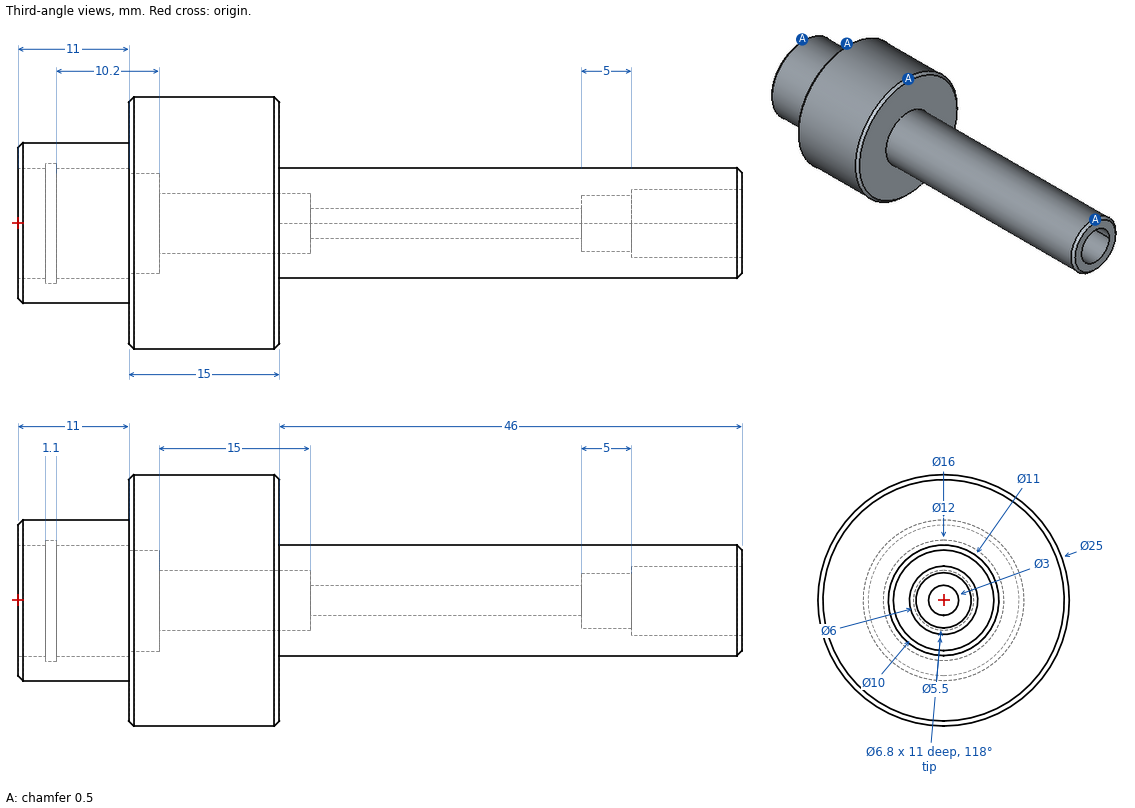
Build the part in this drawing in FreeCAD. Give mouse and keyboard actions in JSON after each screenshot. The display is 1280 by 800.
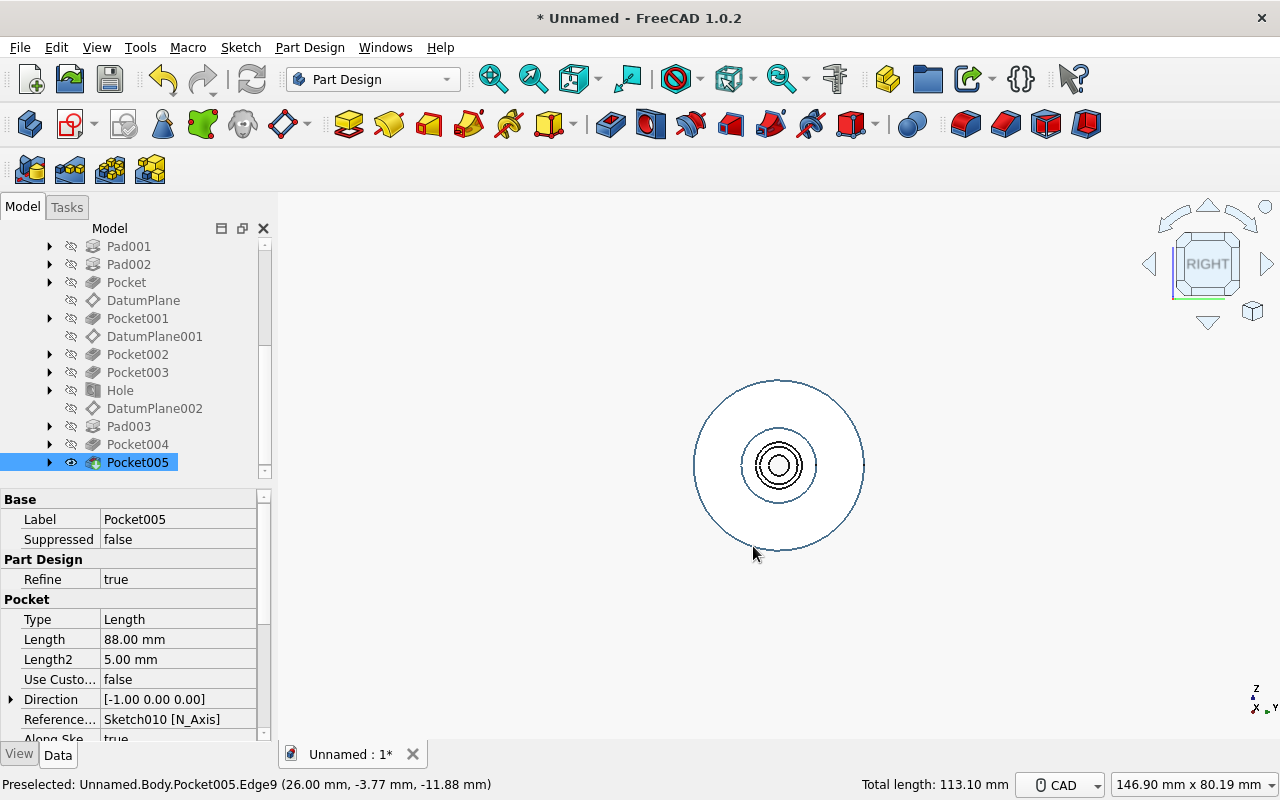
{"action": "key", "text": "0"}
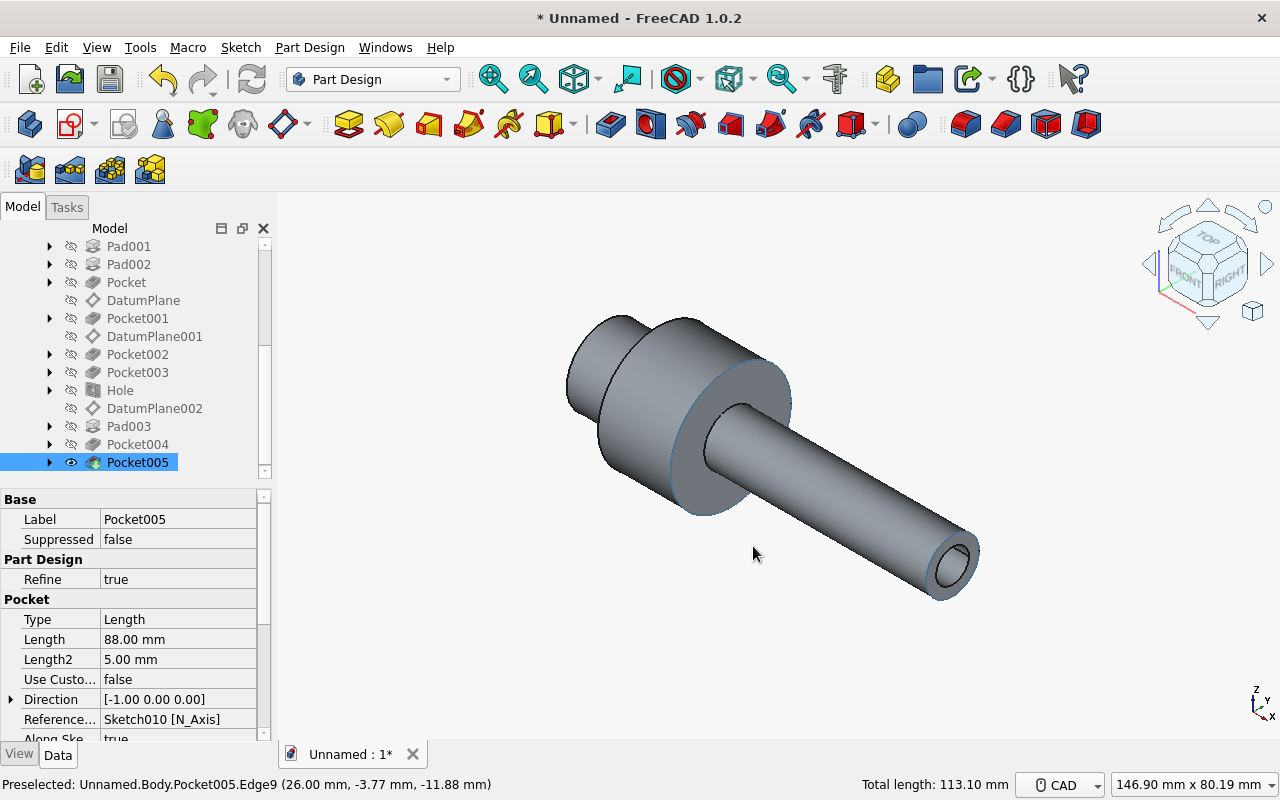
{"action": "left_click", "coordinate": [593, 329], "text": "ctrl"}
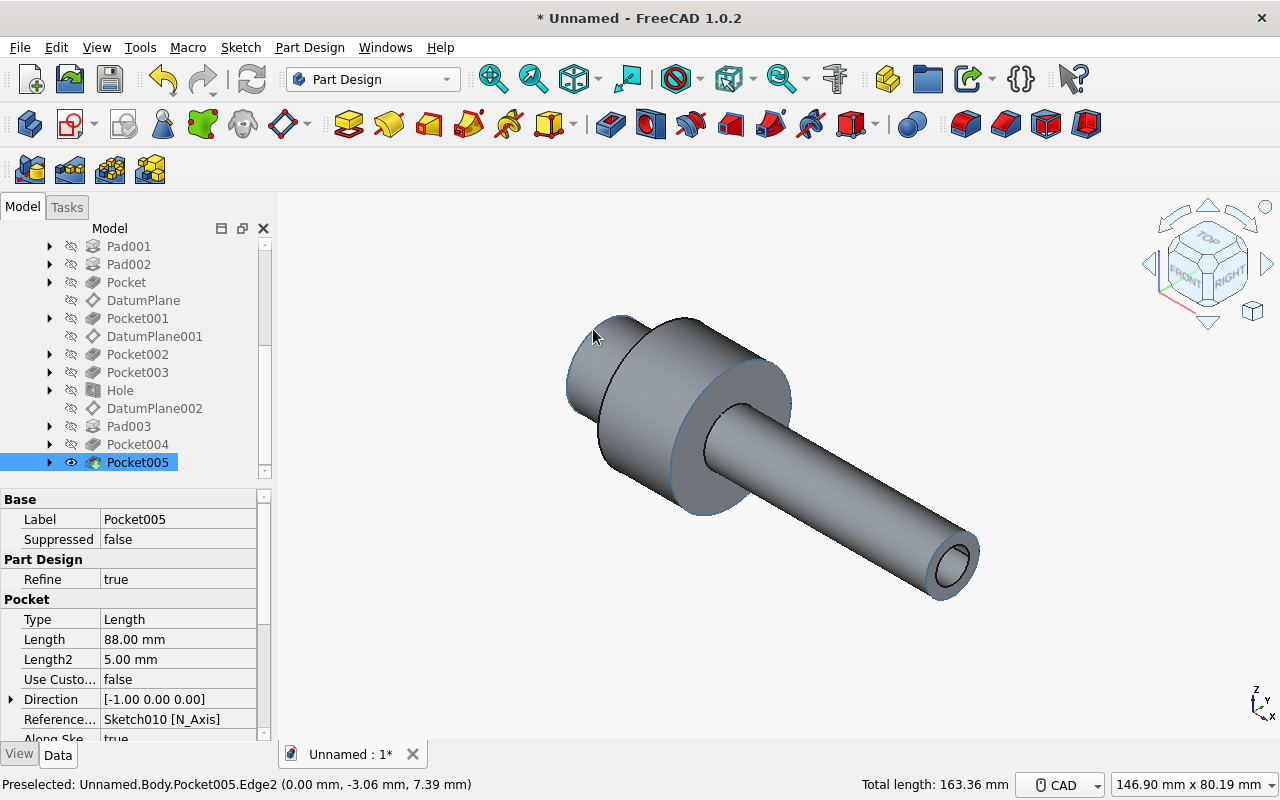
{"action": "left_click", "coordinate": [640, 339], "text": "ctrl"}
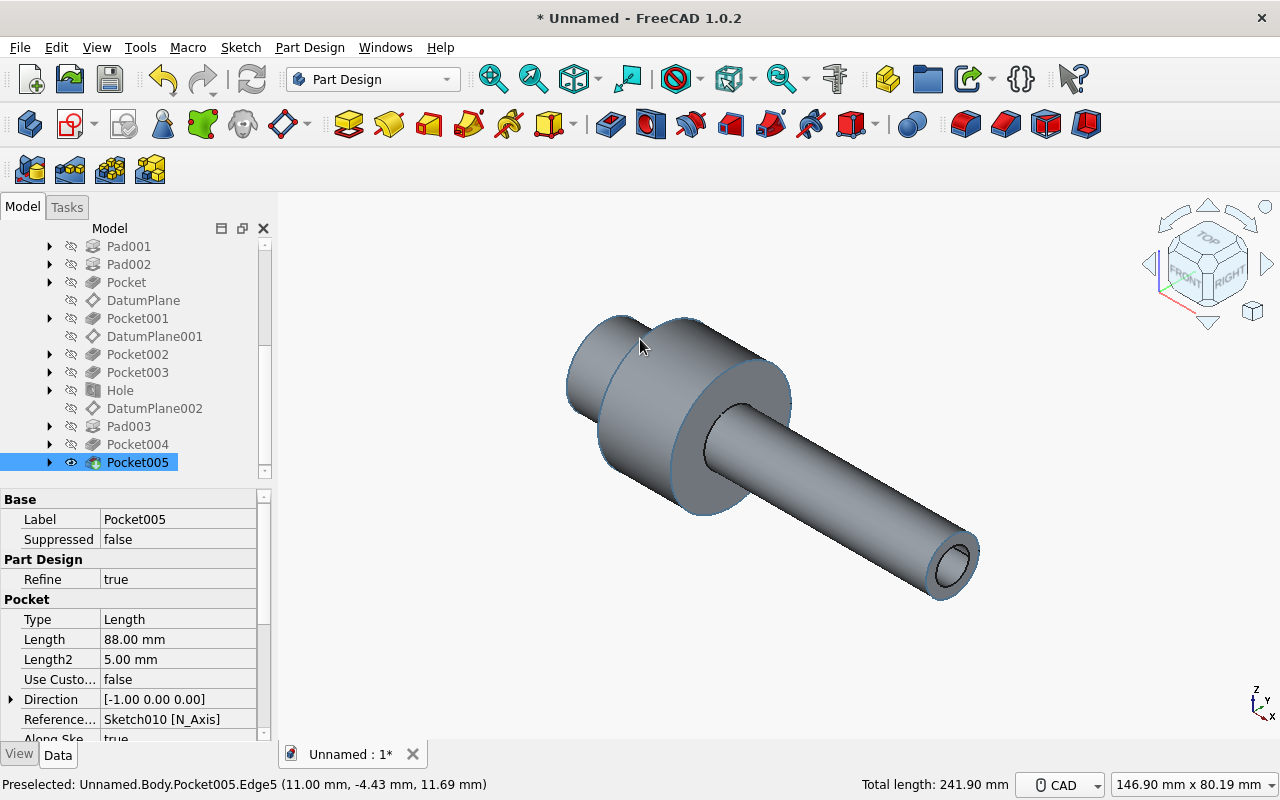
{"action": "left_click", "coordinate": [1006, 124]}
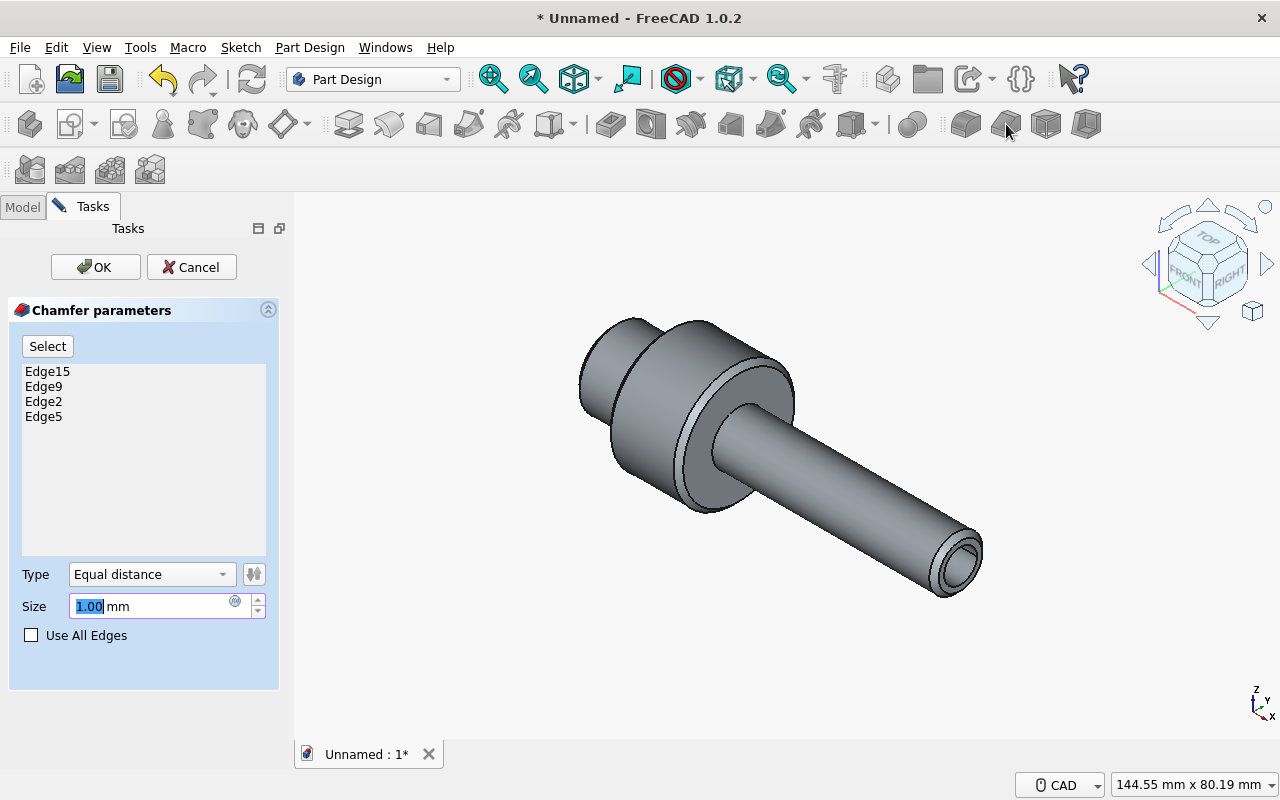
{"action": "type", "text": "0.5"}
{"action": "key", "text": "Tab"}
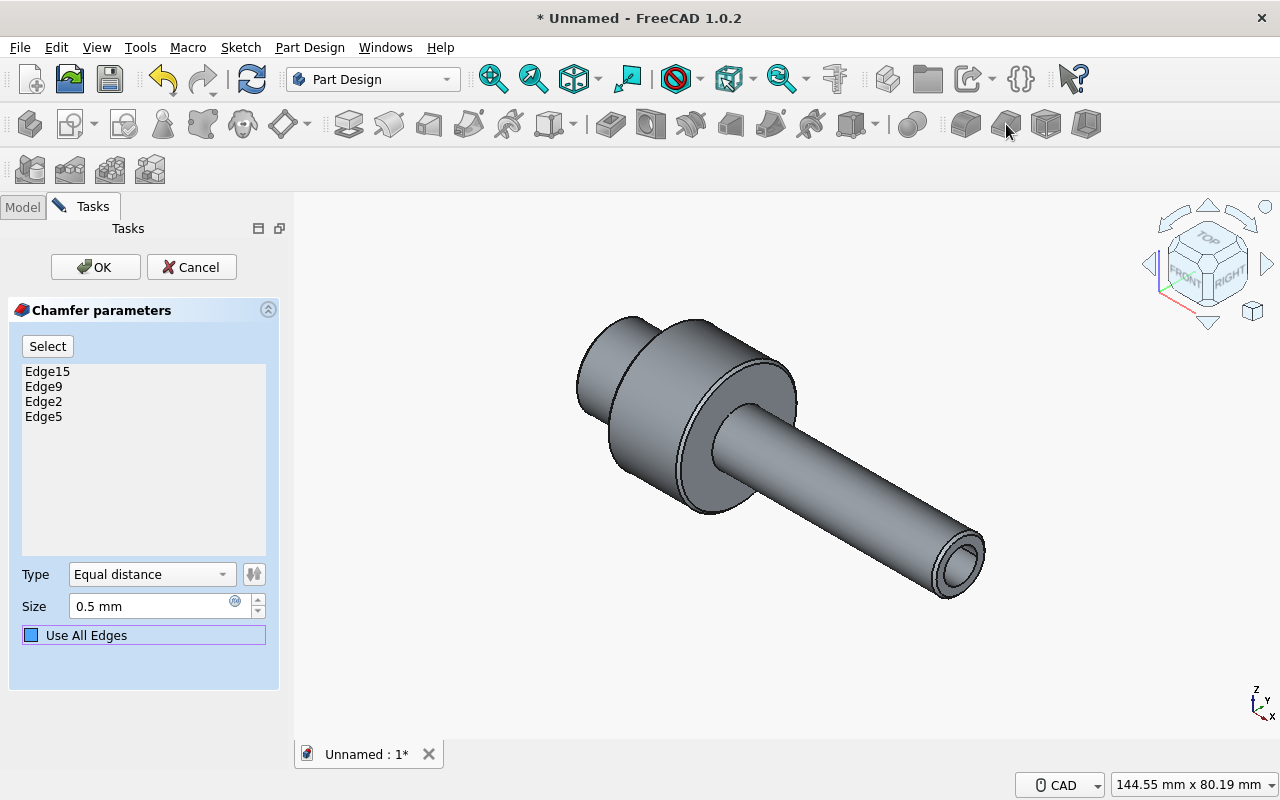
{"action": "left_click", "coordinate": [96, 267]}